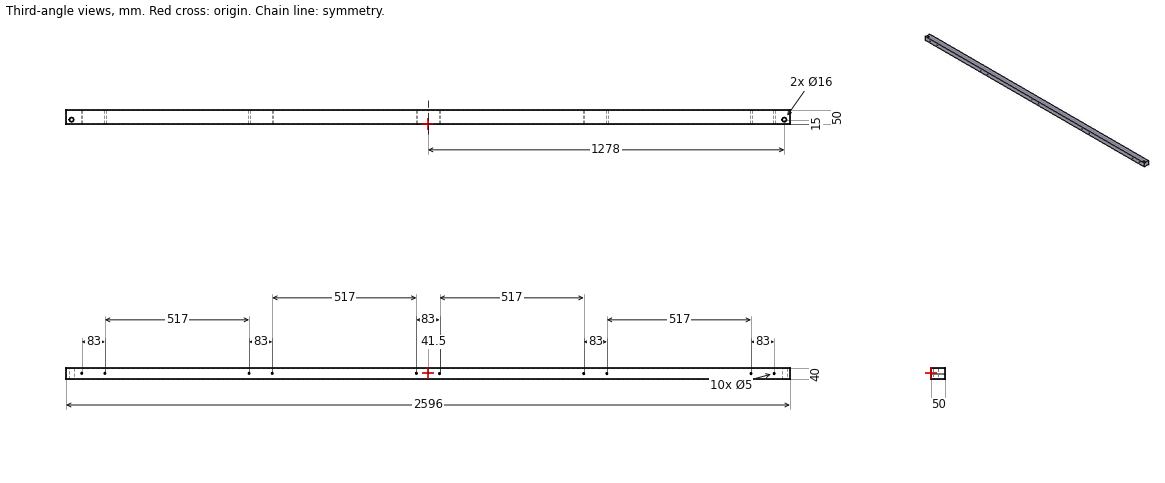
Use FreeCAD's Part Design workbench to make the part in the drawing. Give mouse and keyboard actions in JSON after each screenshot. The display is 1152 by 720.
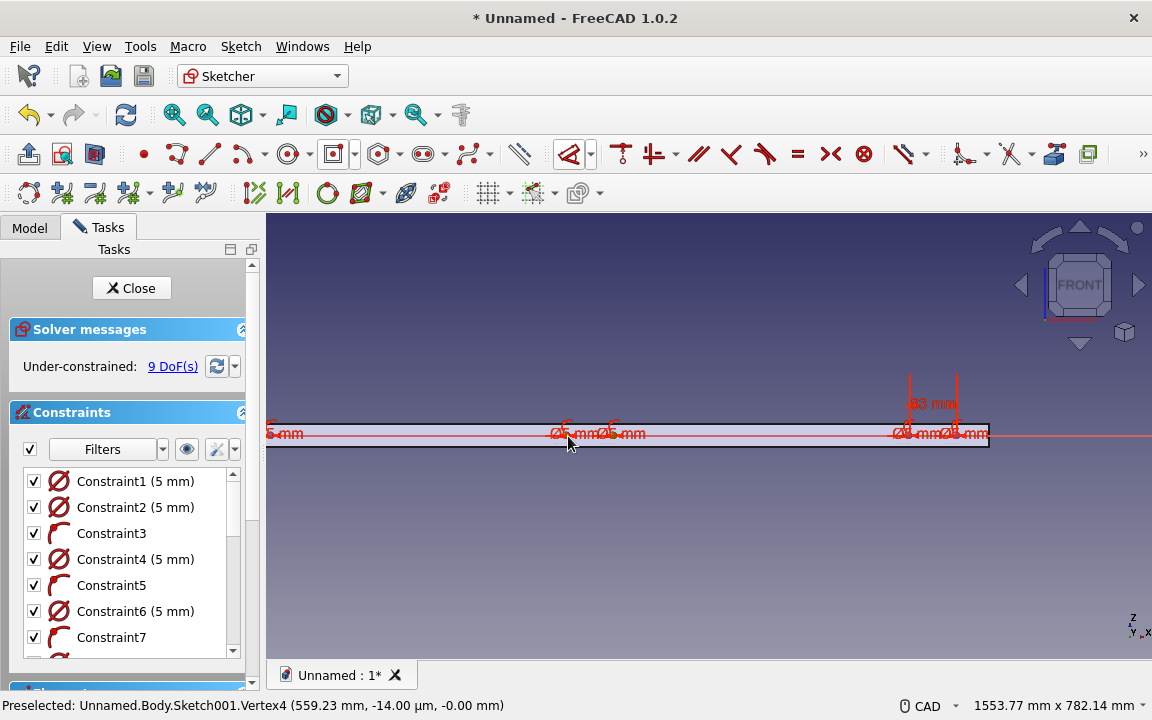
{"action": "left_click", "coordinate": [590, 154]}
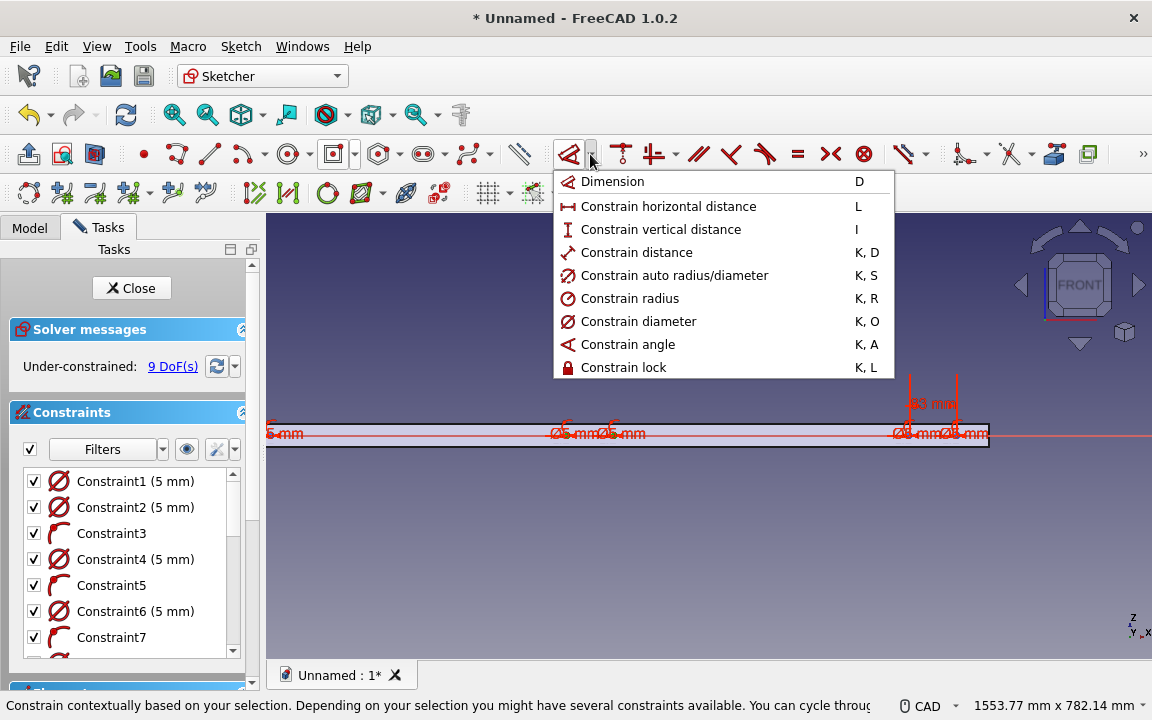
{"action": "left_click", "coordinate": [724, 206]}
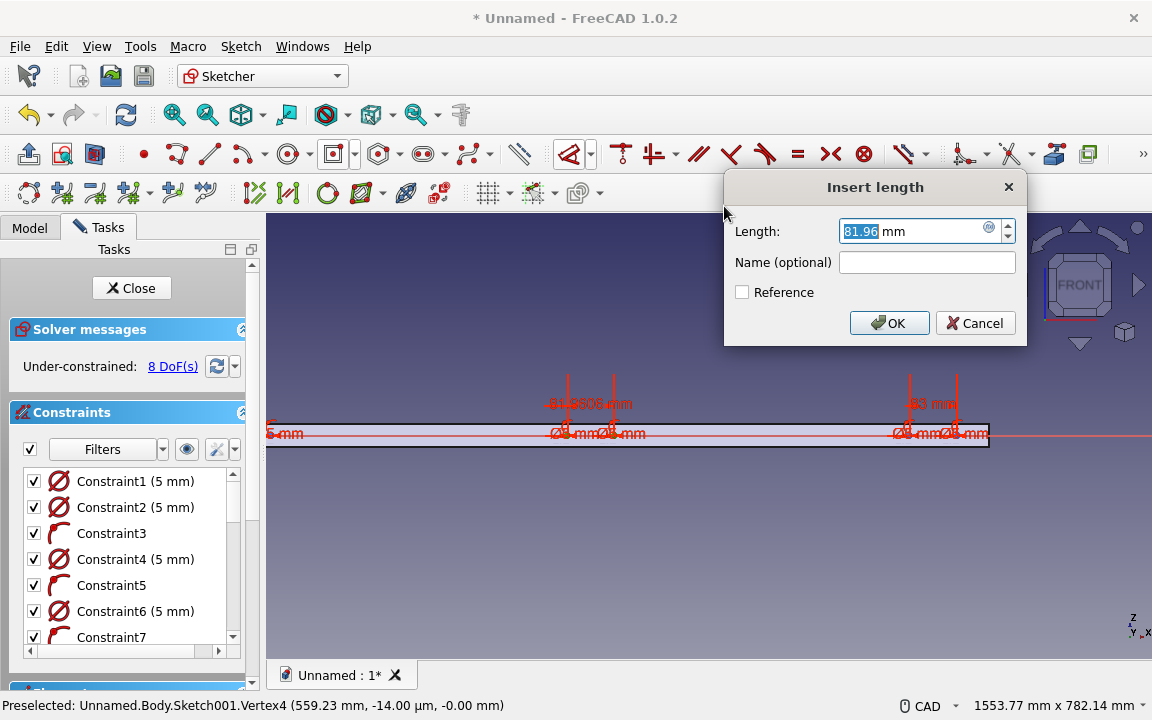
{"action": "type", "text": "83"}
{"action": "key", "text": "Return"}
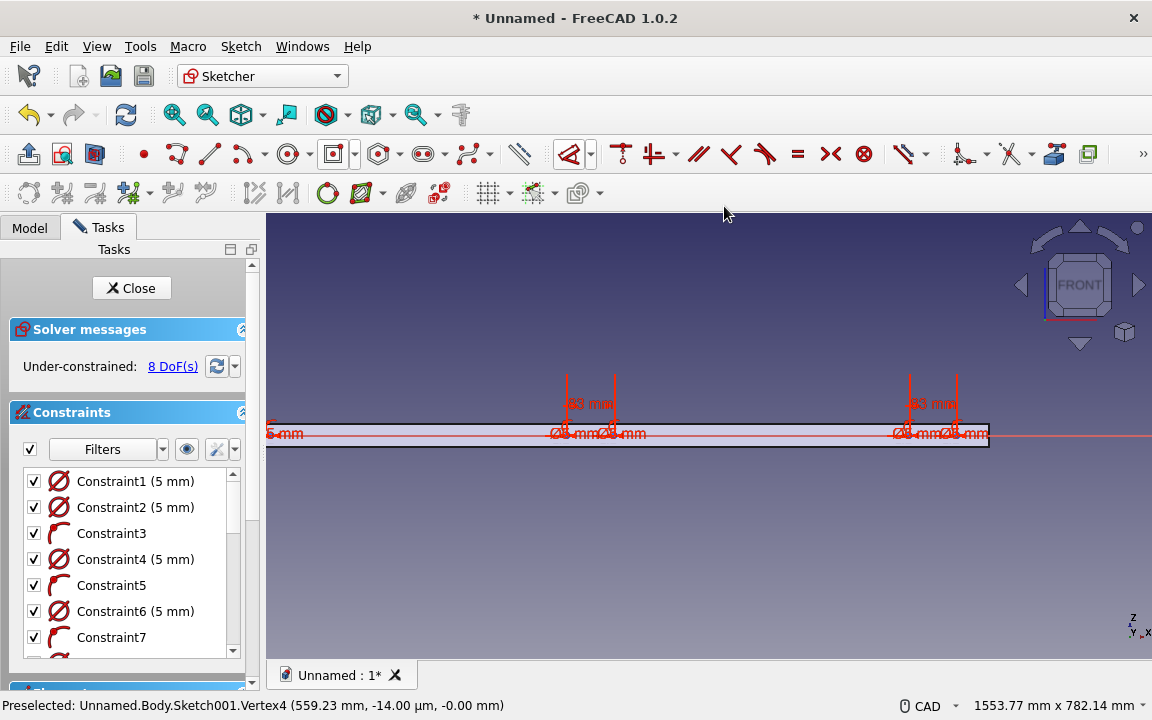
{"action": "scroll", "coordinate": [869, 436], "scroll_direction": "down", "scroll_amount": 5}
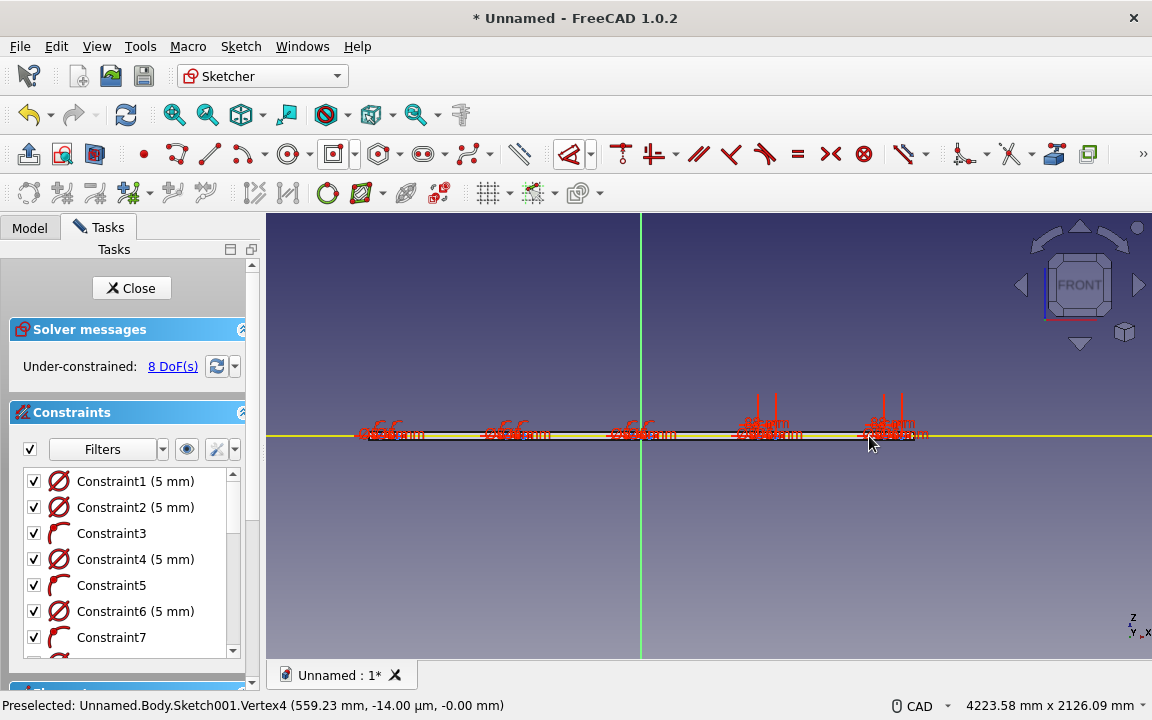
{"action": "scroll", "coordinate": [650, 436], "scroll_direction": "up", "scroll_amount": 5}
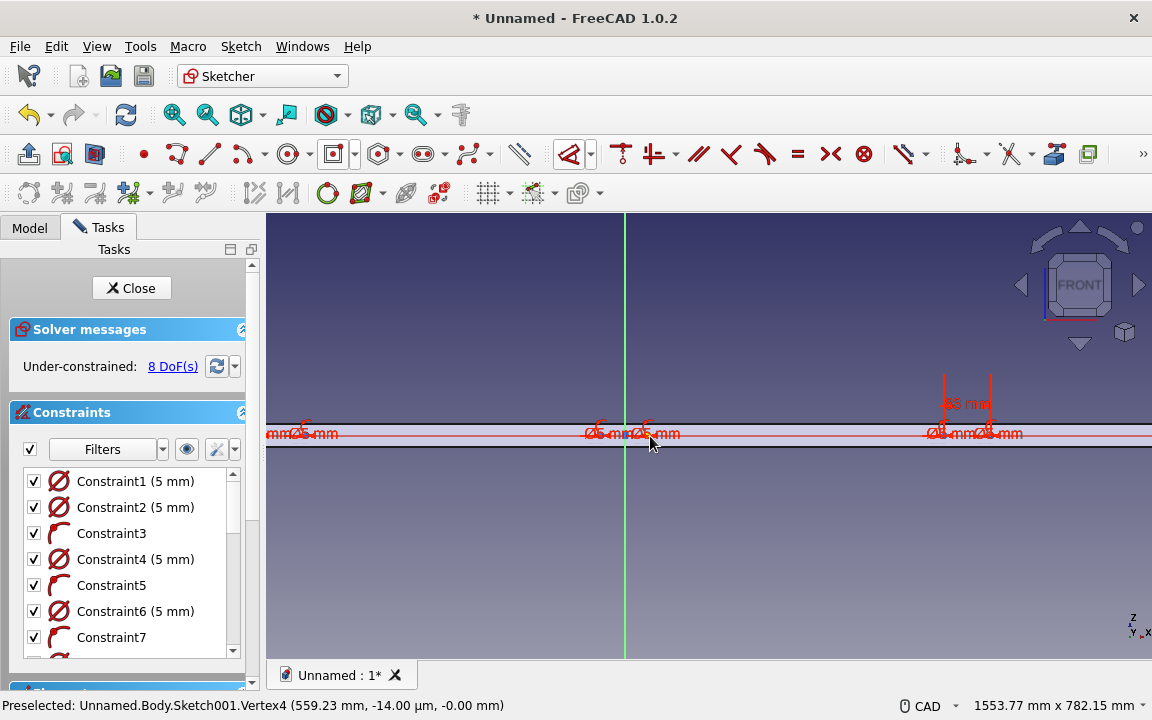
{"action": "left_click", "coordinate": [649, 436]}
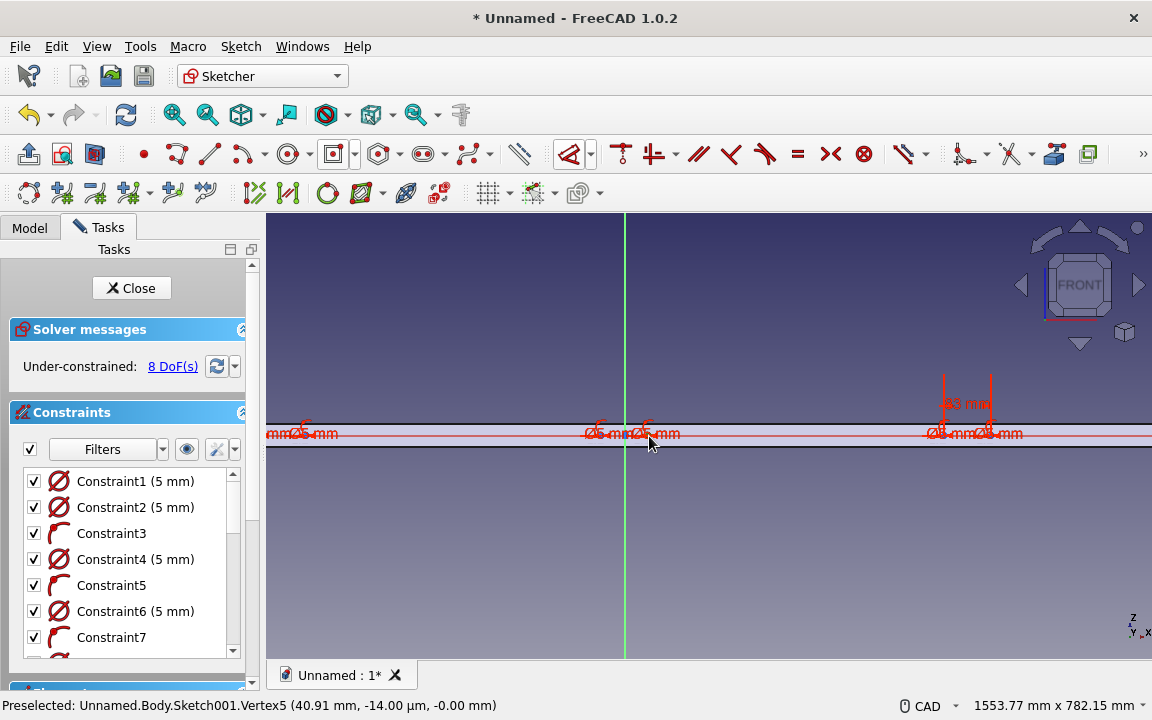
{"action": "left_click", "coordinate": [602, 436]}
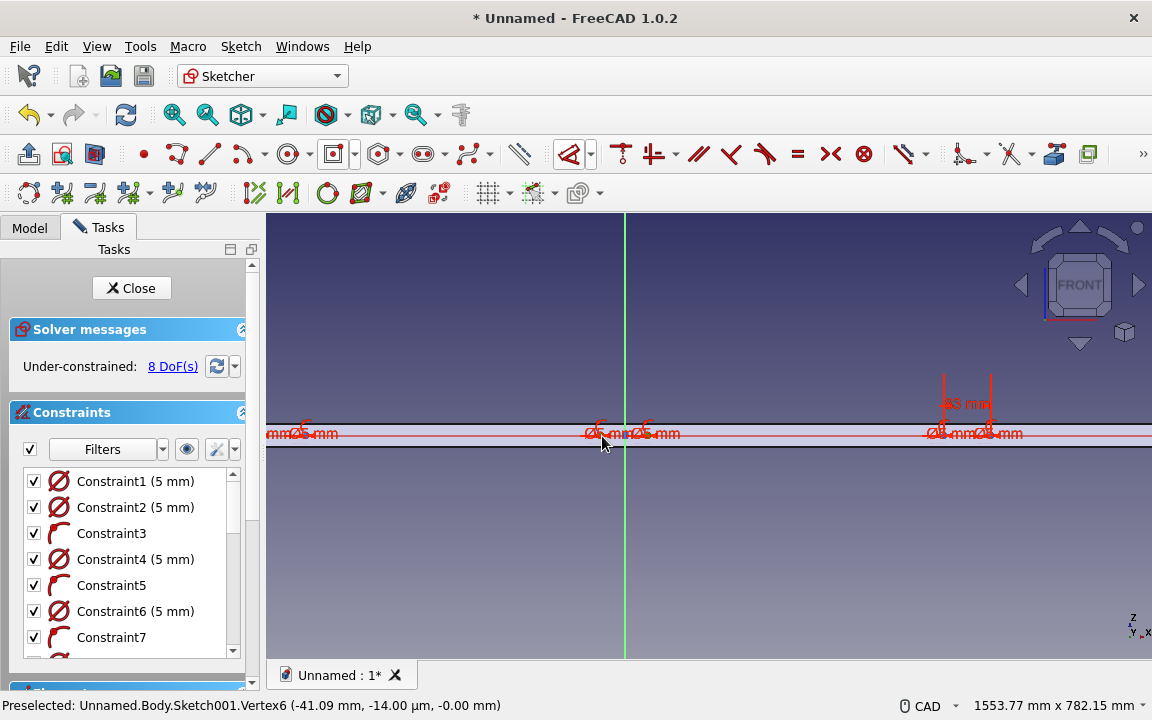
{"action": "left_click", "coordinate": [590, 154]}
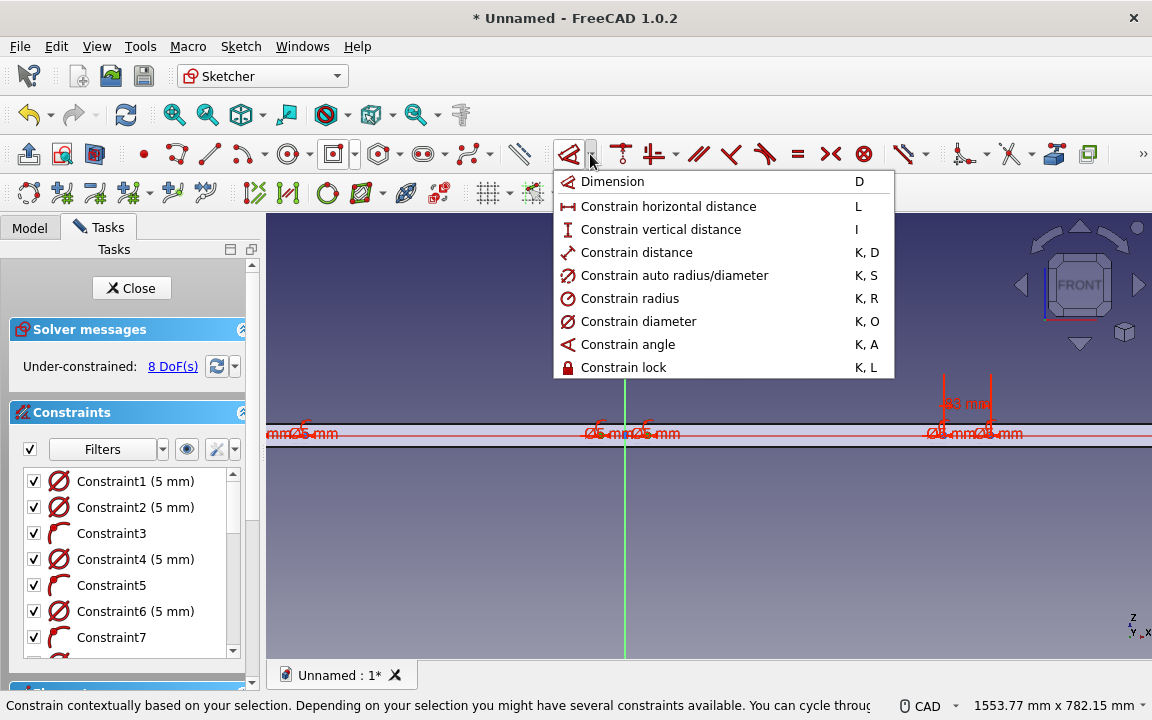
{"action": "left_click", "coordinate": [724, 206]}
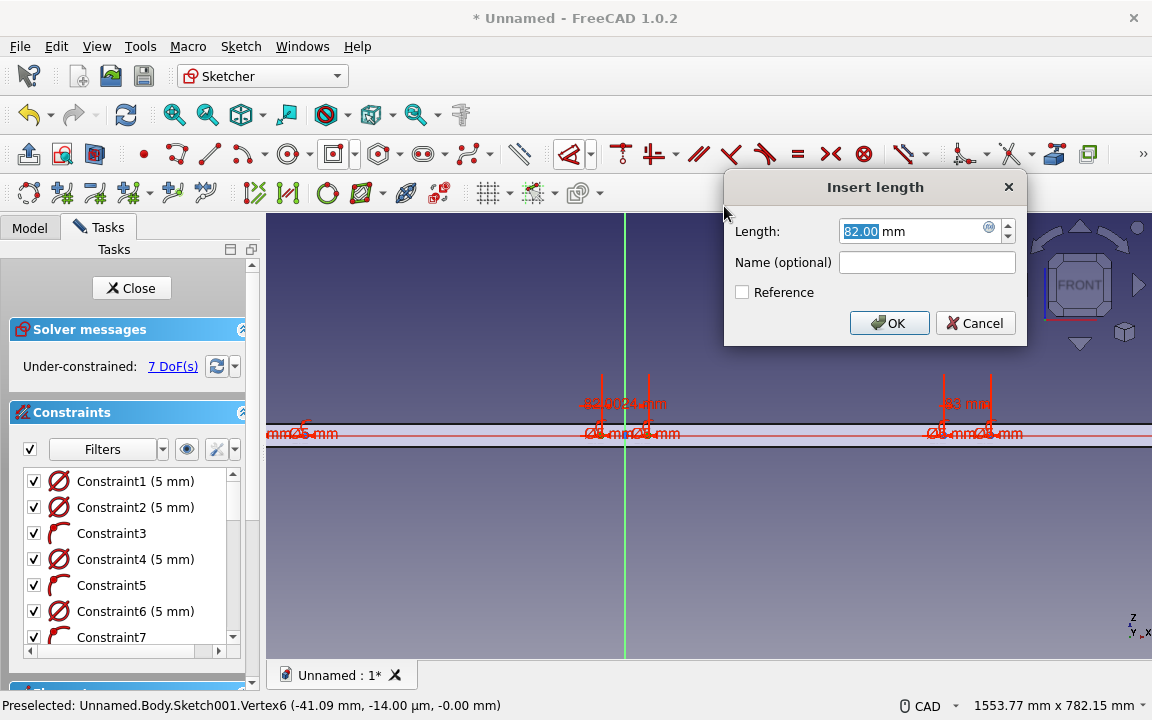
{"action": "type", "text": "83"}
{"action": "key", "text": "Return"}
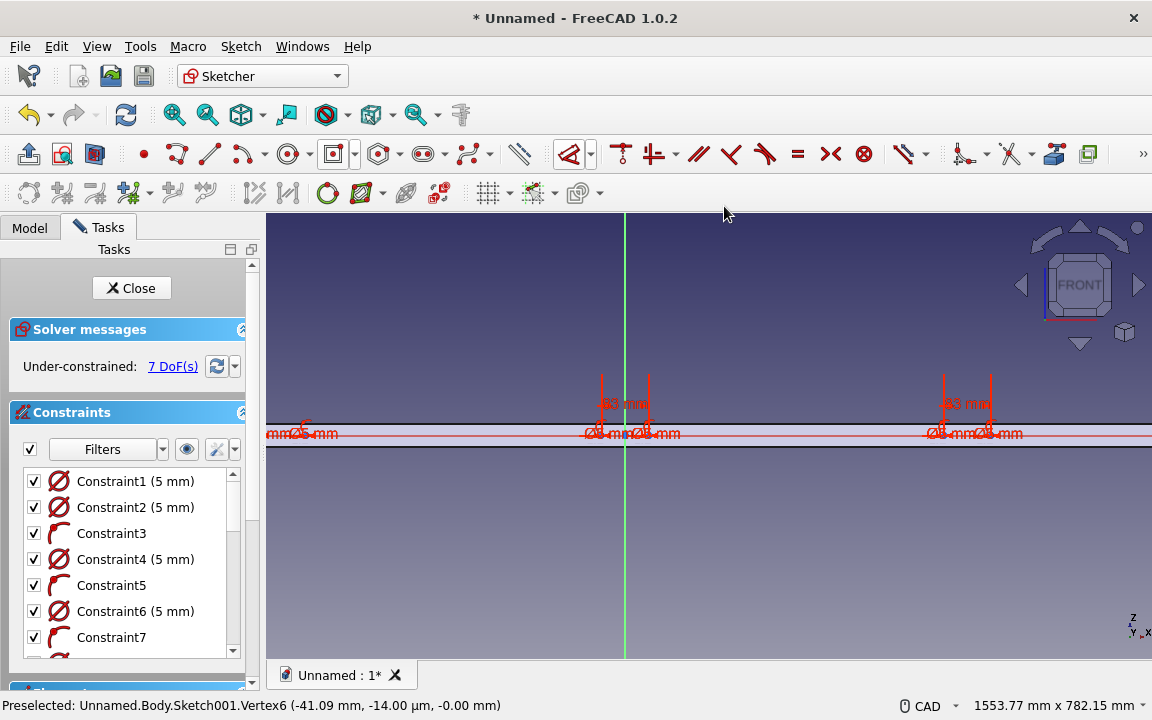
{"action": "left_click", "coordinate": [307, 436]}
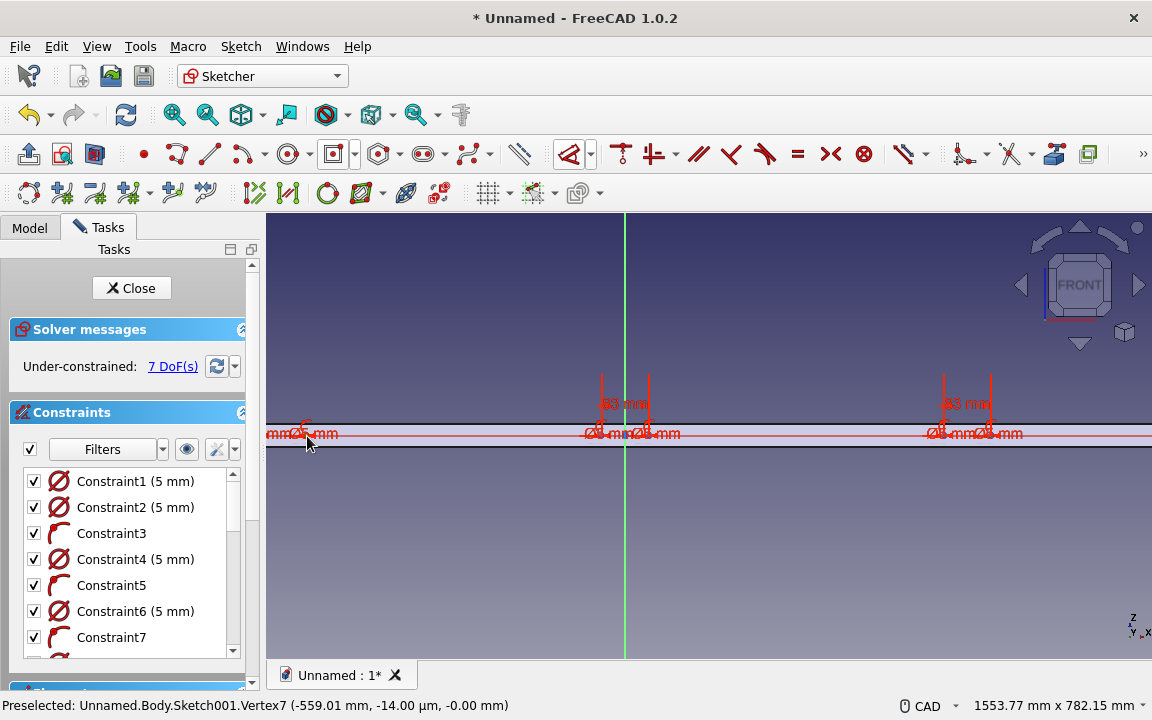
{"action": "scroll", "coordinate": [649, 436], "scroll_direction": "down", "scroll_amount": 5}